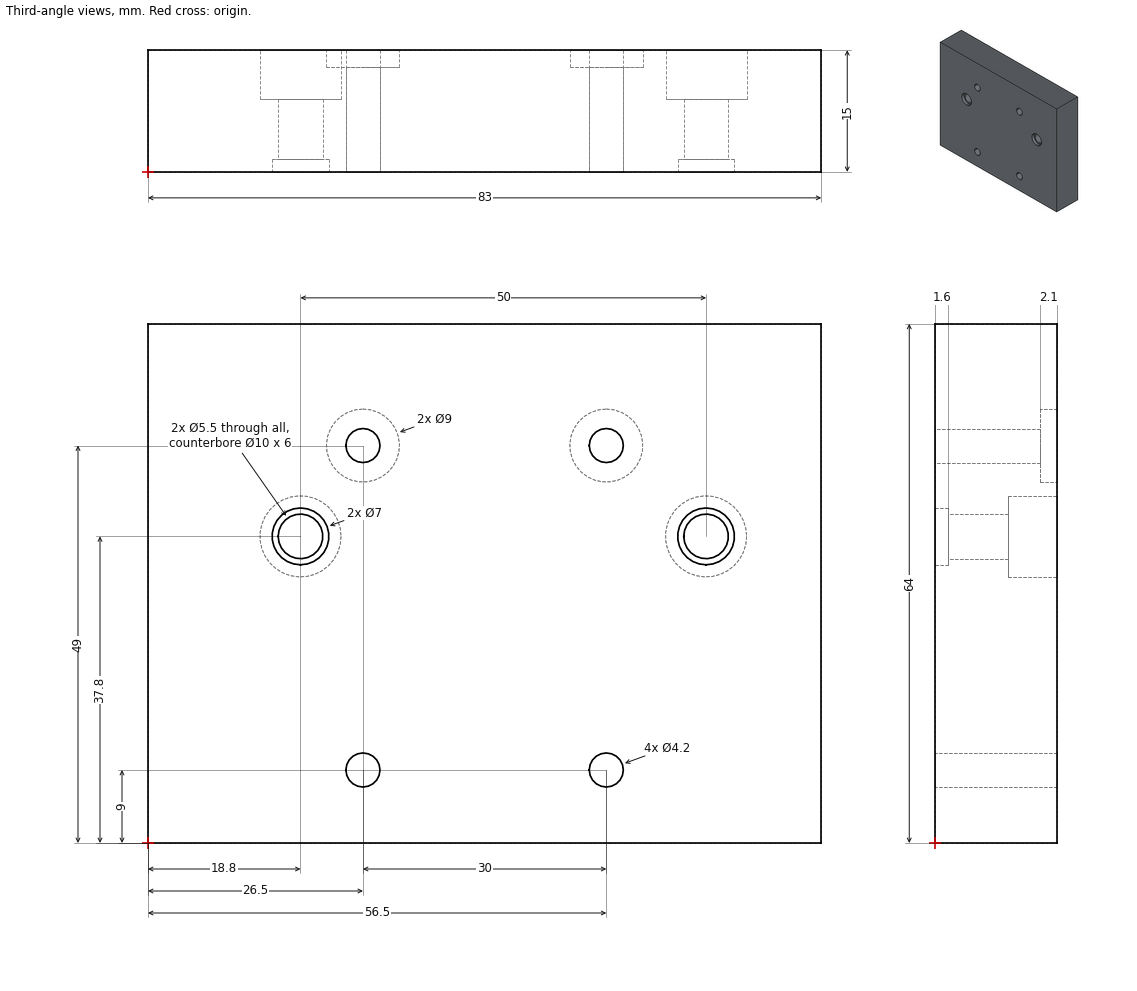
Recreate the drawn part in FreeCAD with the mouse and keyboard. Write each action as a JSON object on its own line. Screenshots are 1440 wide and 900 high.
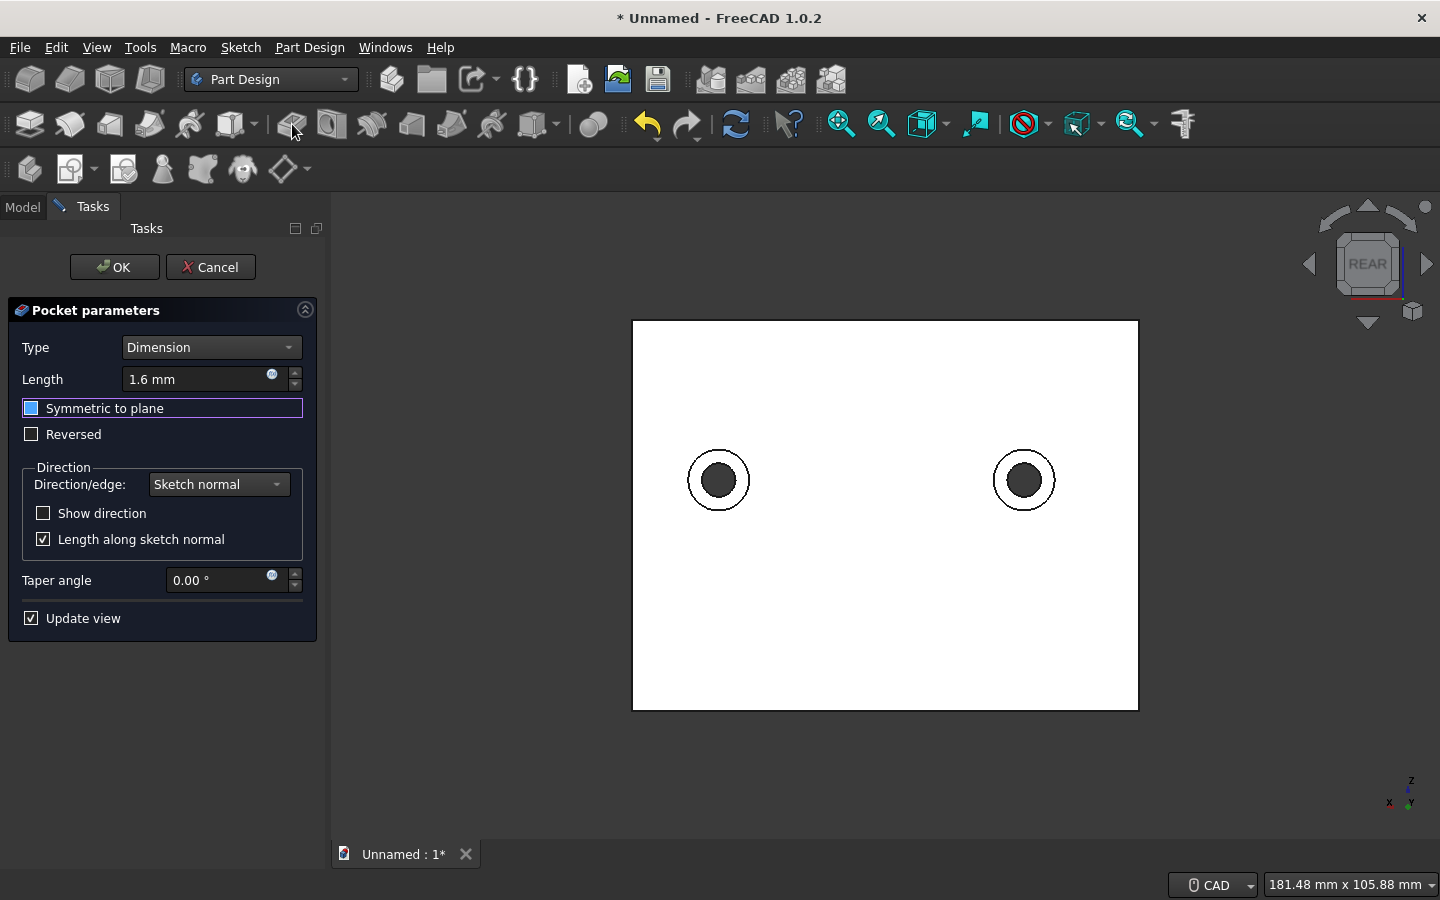
{"action": "left_click", "coordinate": [115, 267]}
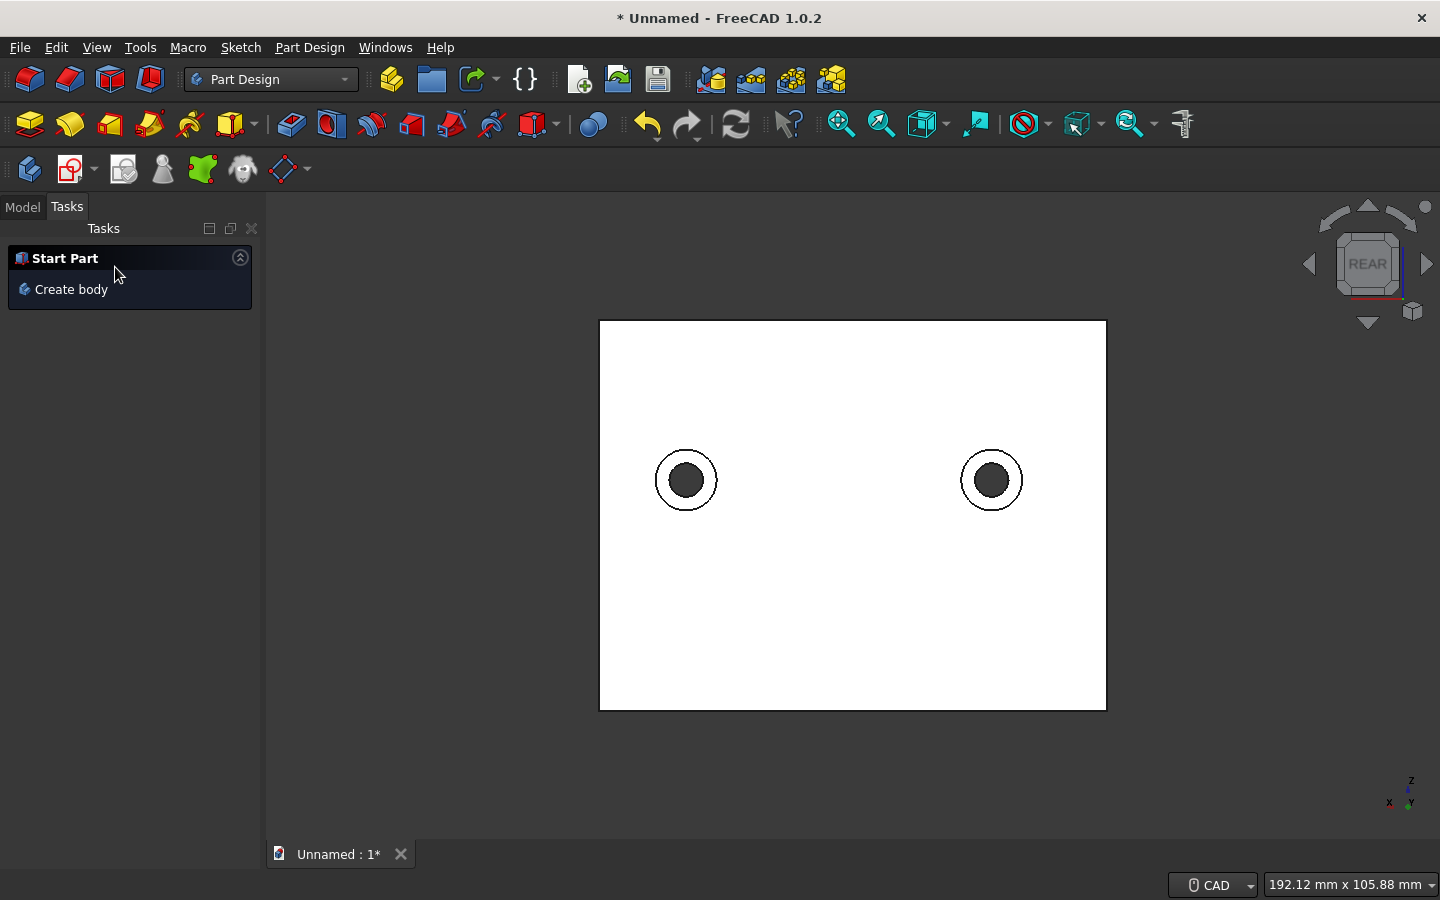
{"action": "left_click", "coordinate": [853, 570]}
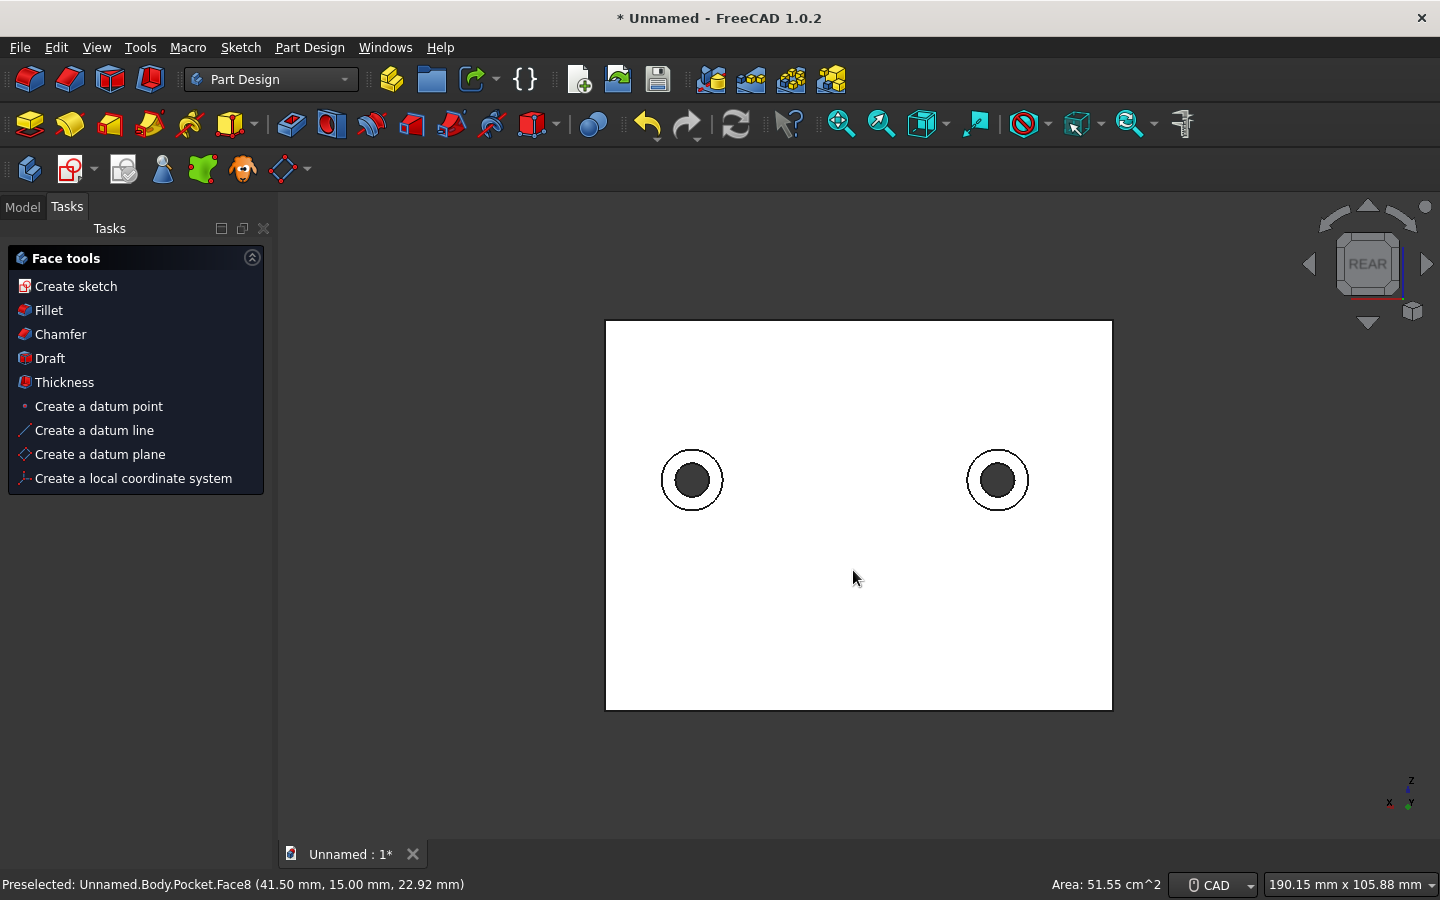
{"action": "left_click", "coordinate": [70, 170]}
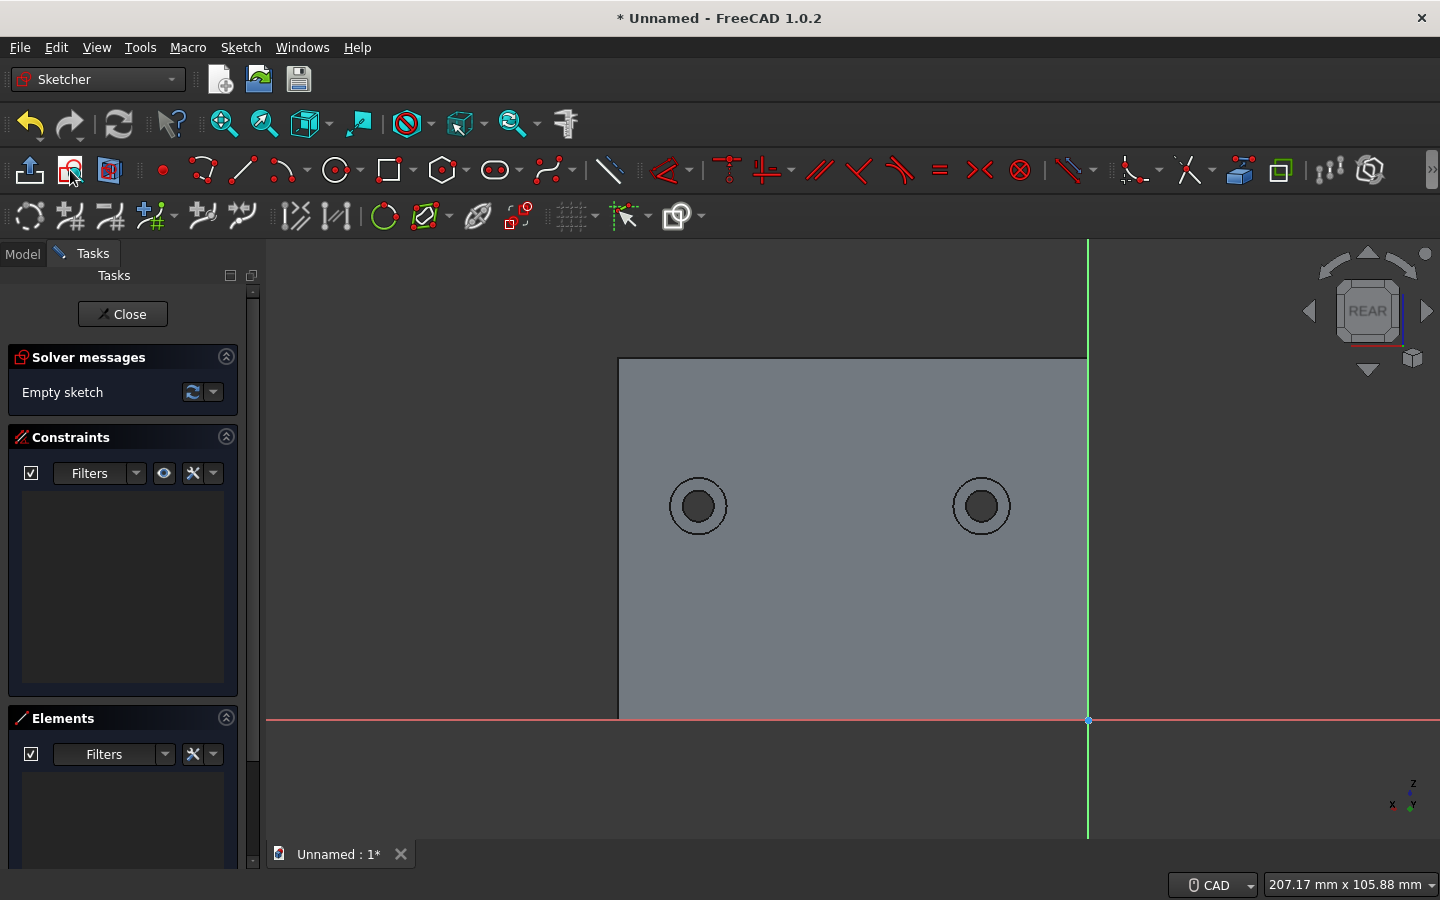
{"action": "left_click", "coordinate": [336, 170]}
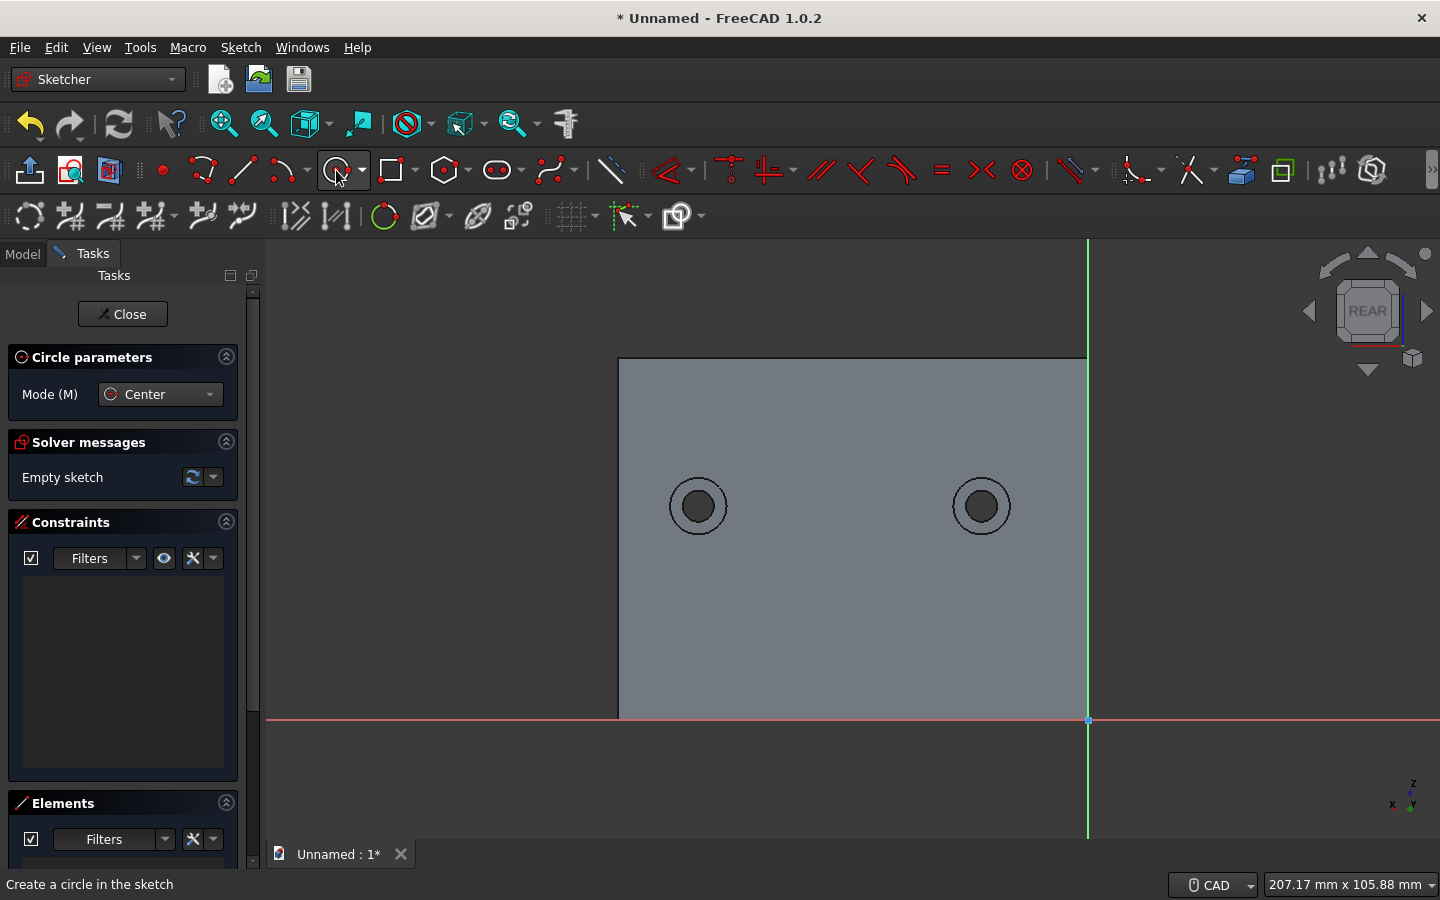
{"action": "scroll", "coordinate": [768, 669], "scroll_direction": "up", "scroll_amount": 4}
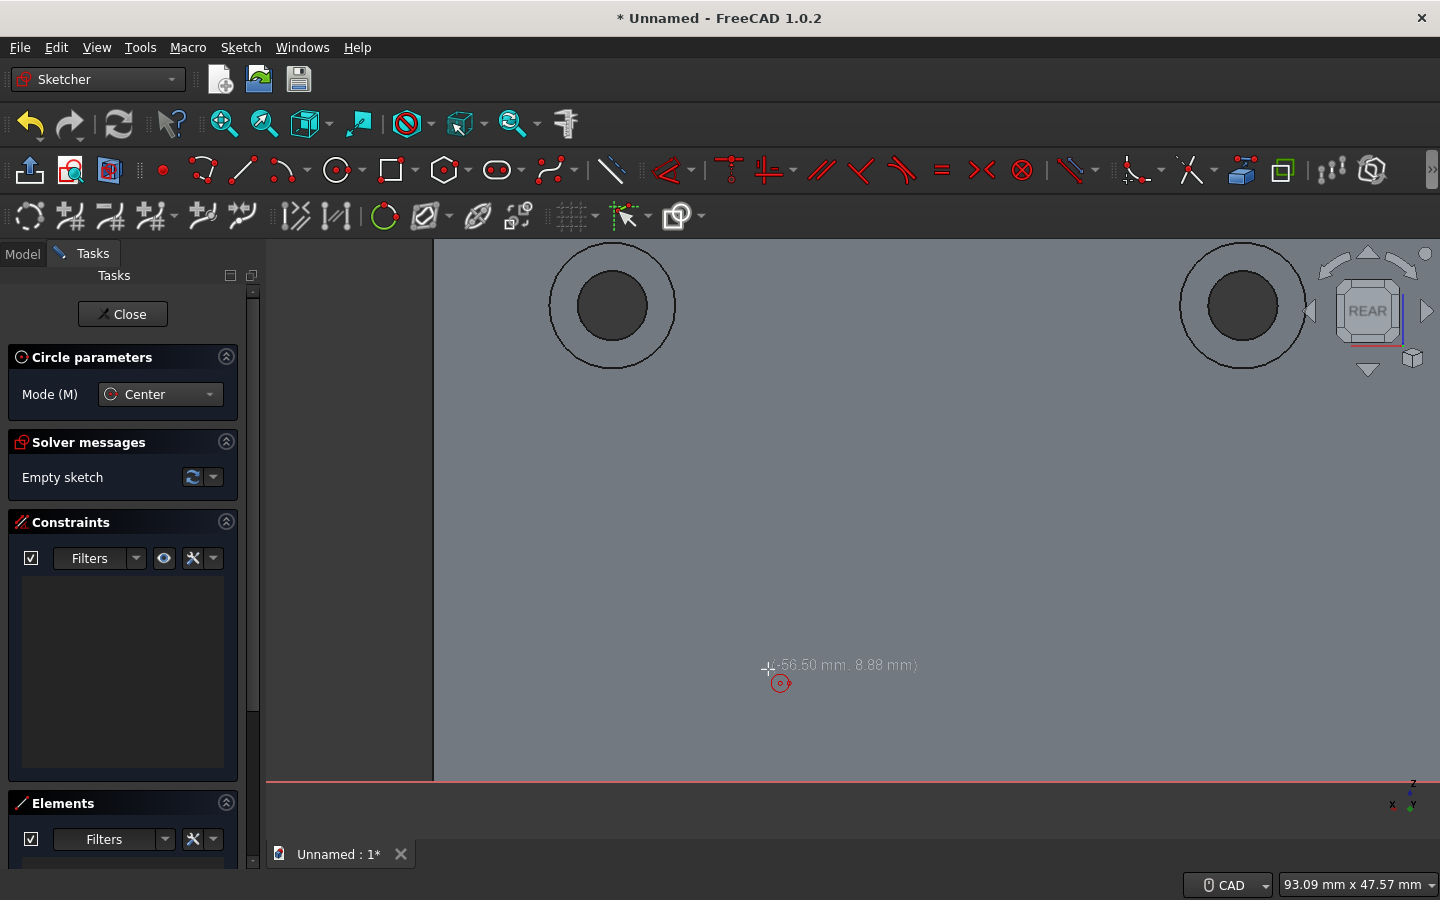
{"action": "left_click", "coordinate": [767, 669]}
{"action": "left_click", "coordinate": [786, 650]}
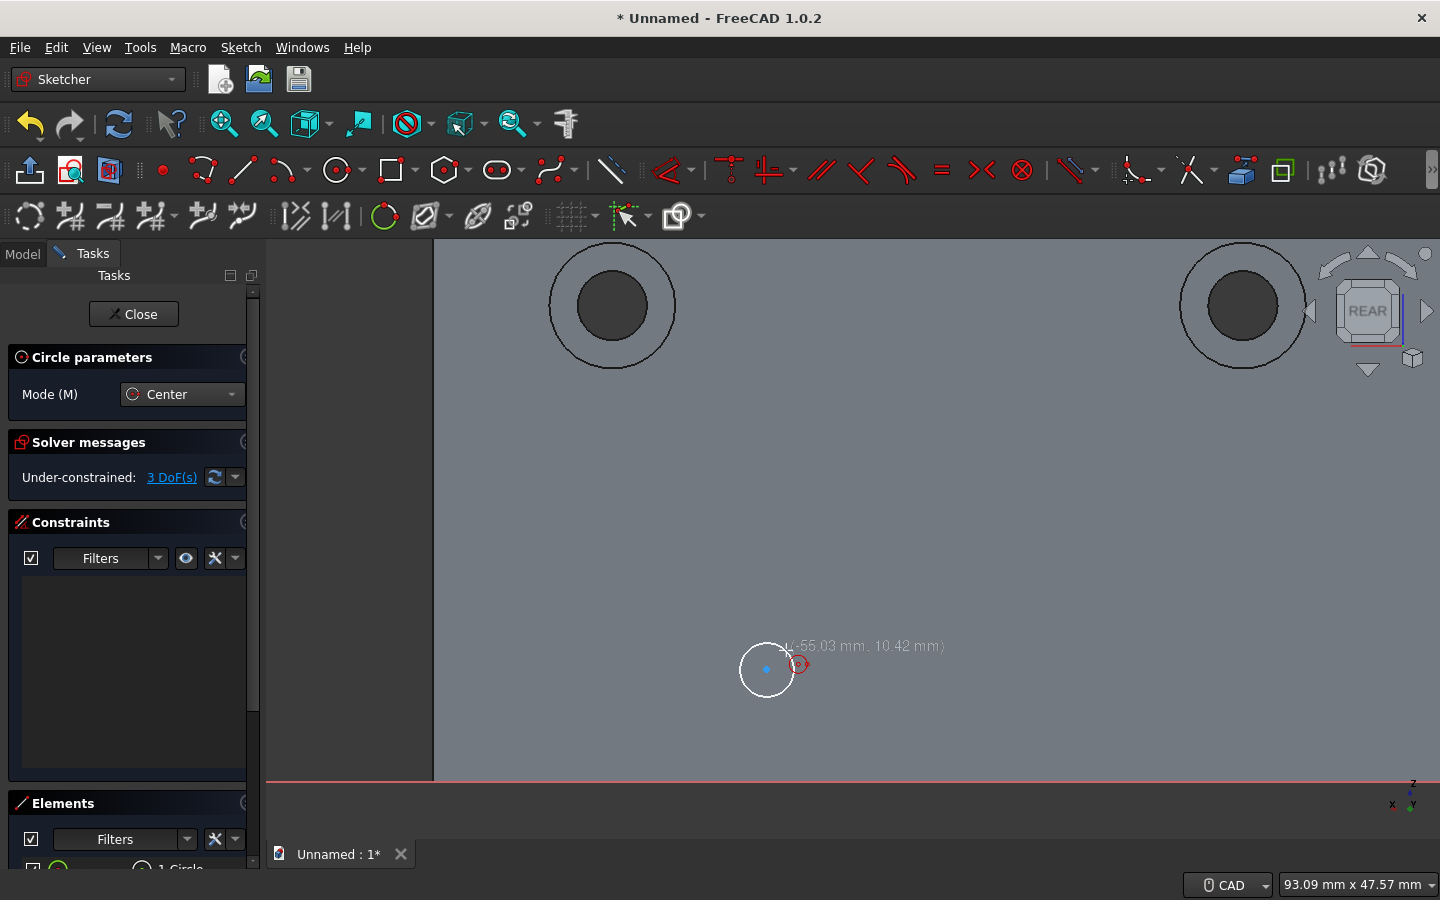
{"action": "left_click", "coordinate": [1146, 669]}
{"action": "left_click", "coordinate": [1165, 650]}